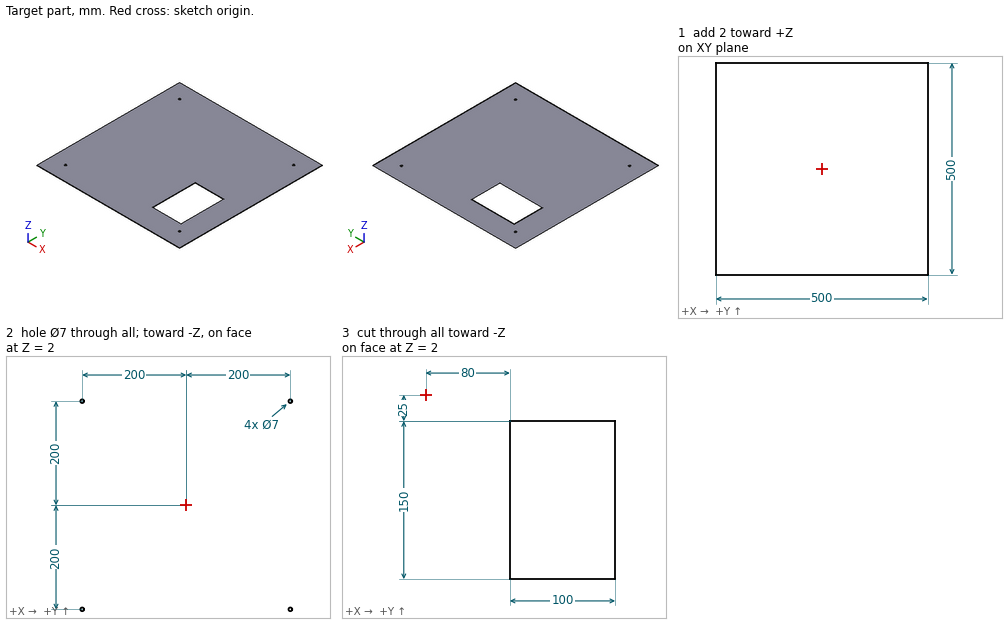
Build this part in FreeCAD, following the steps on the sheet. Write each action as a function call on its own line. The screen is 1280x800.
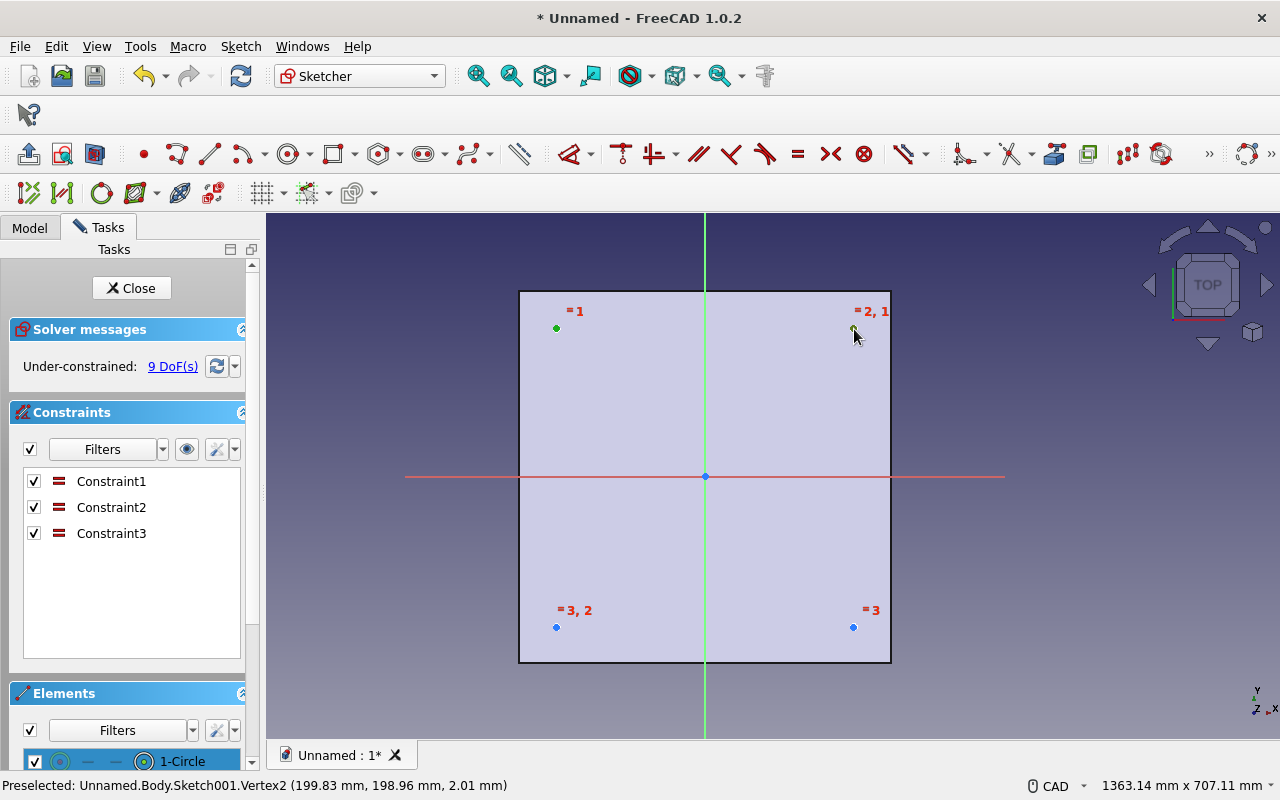
key(h)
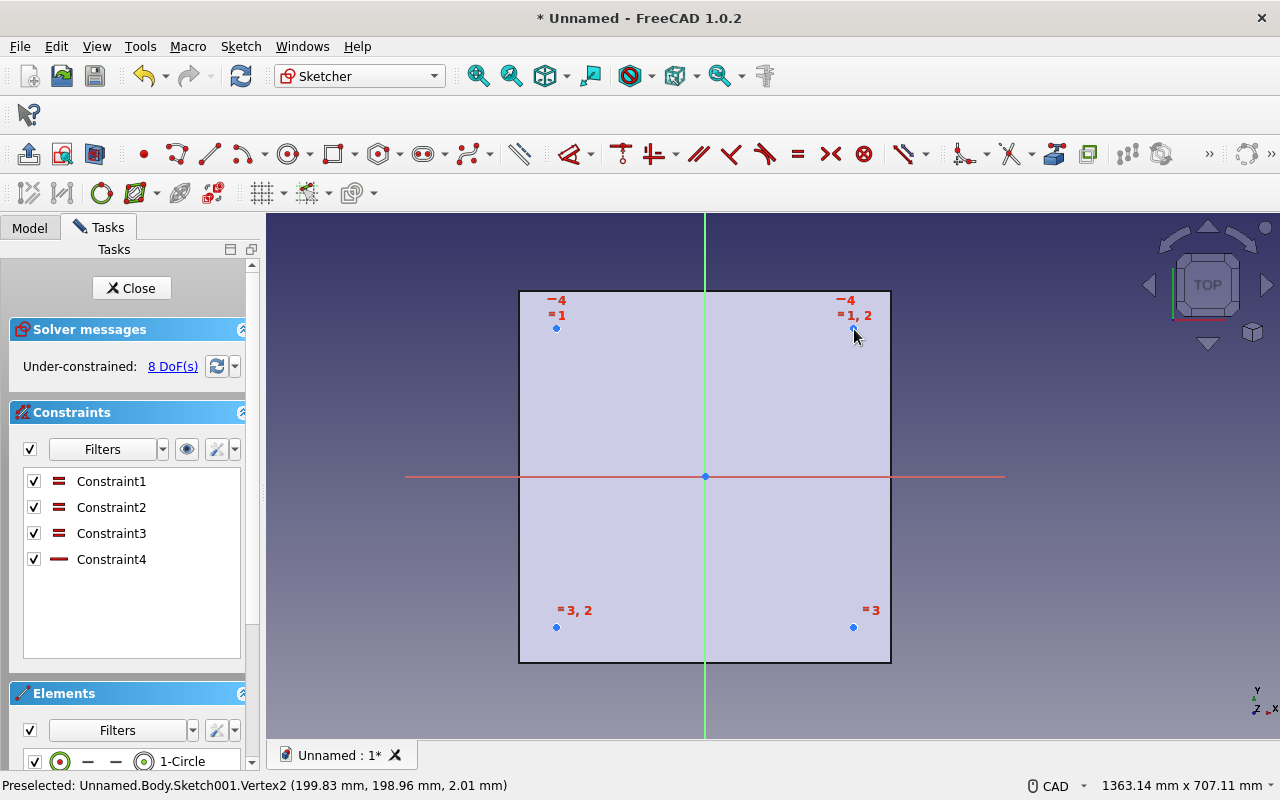
click(557, 329)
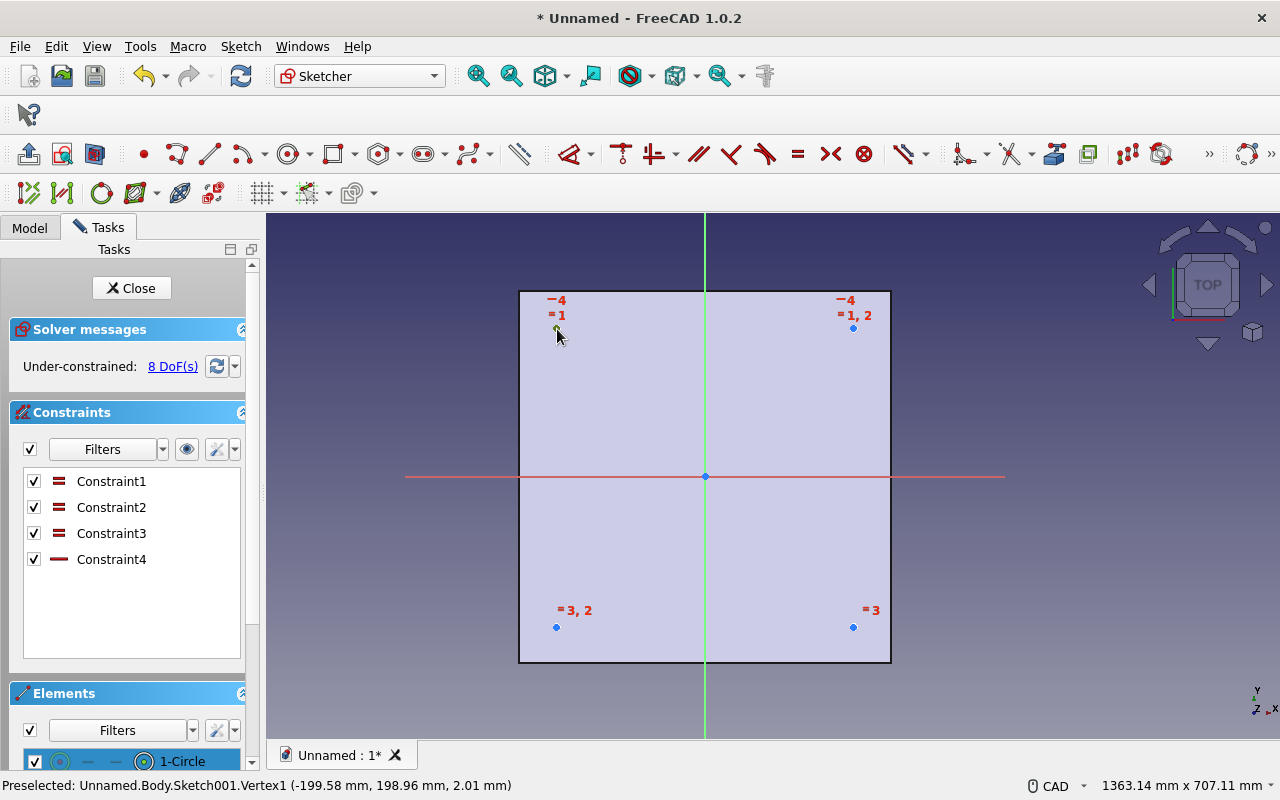
click(557, 627)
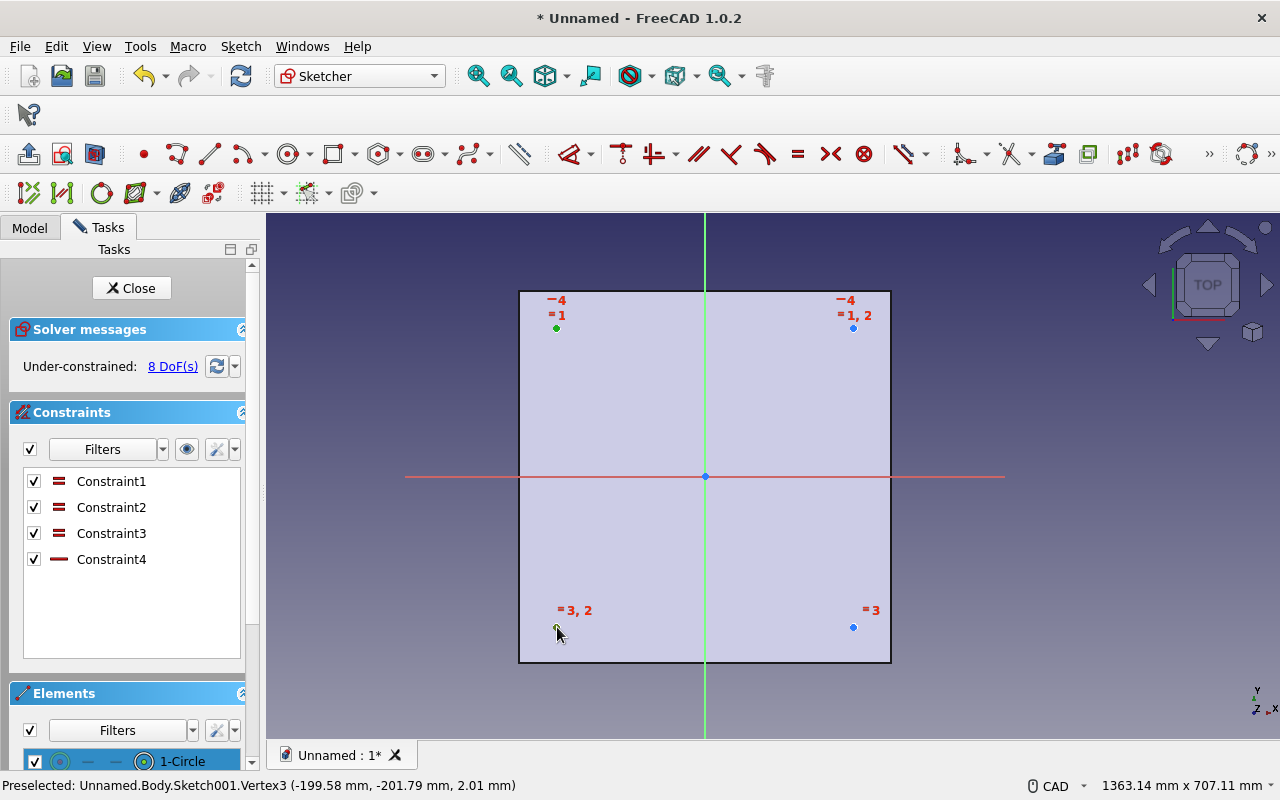
key(v)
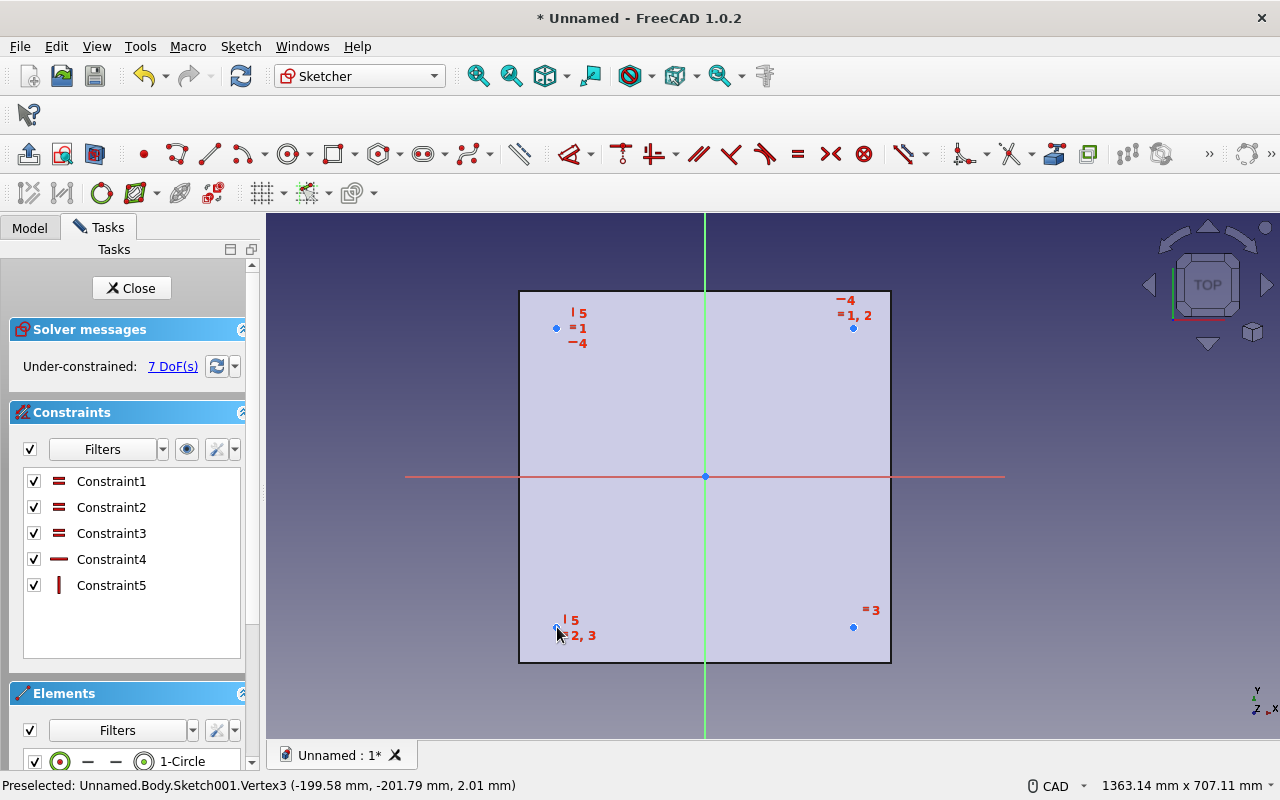
click(854, 329)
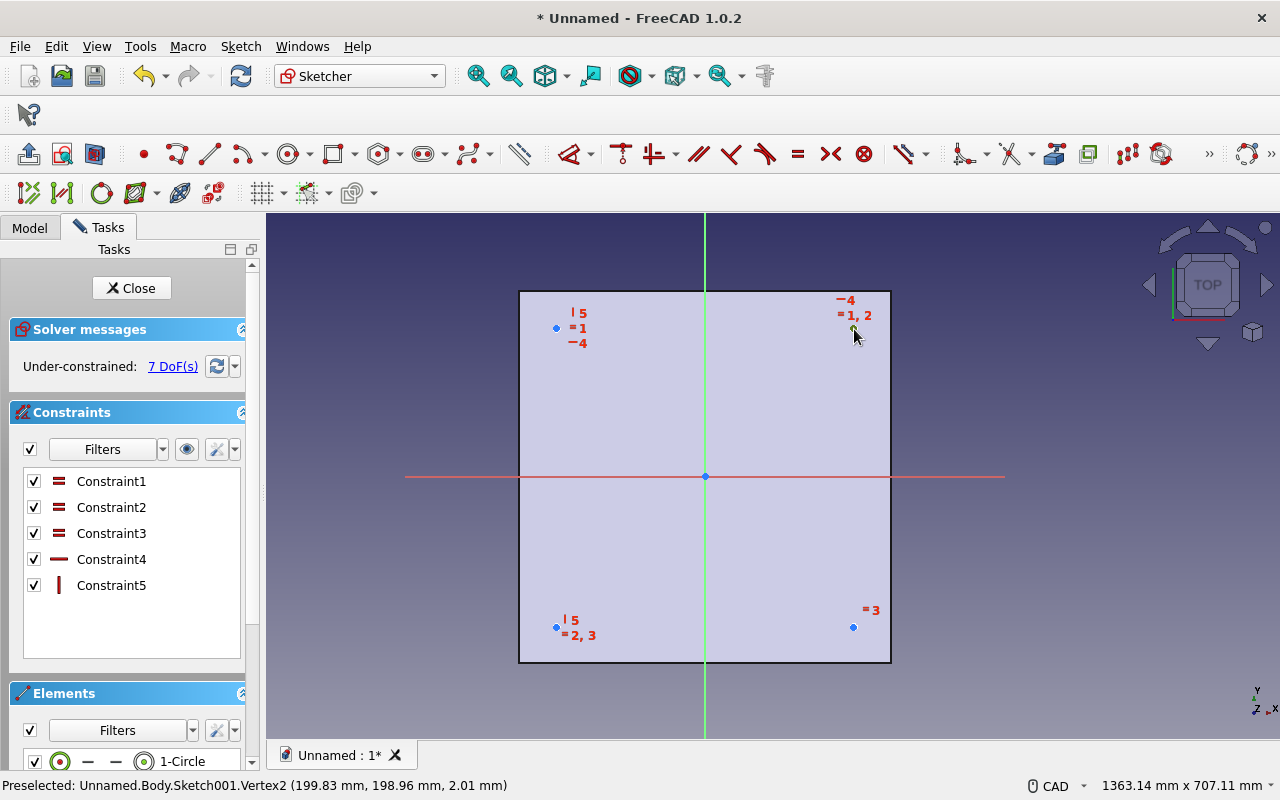
click(854, 627)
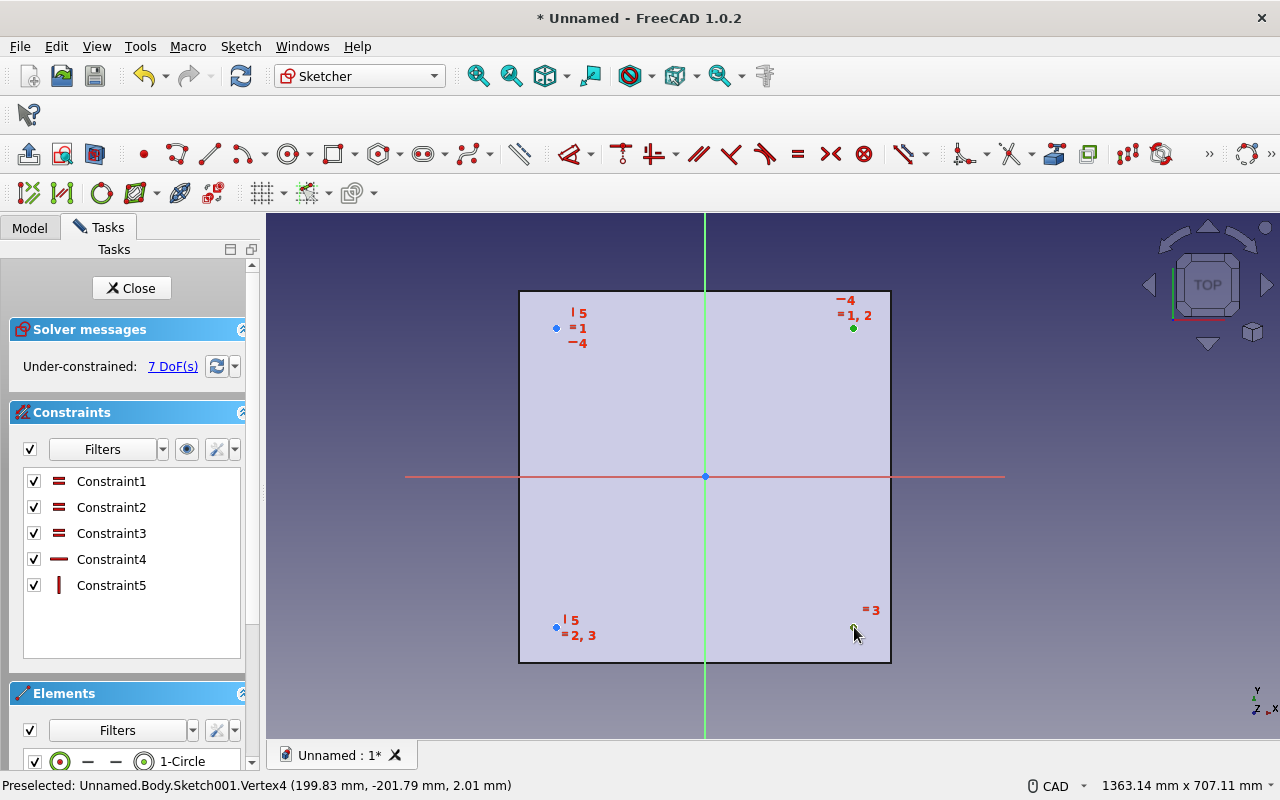
key(v)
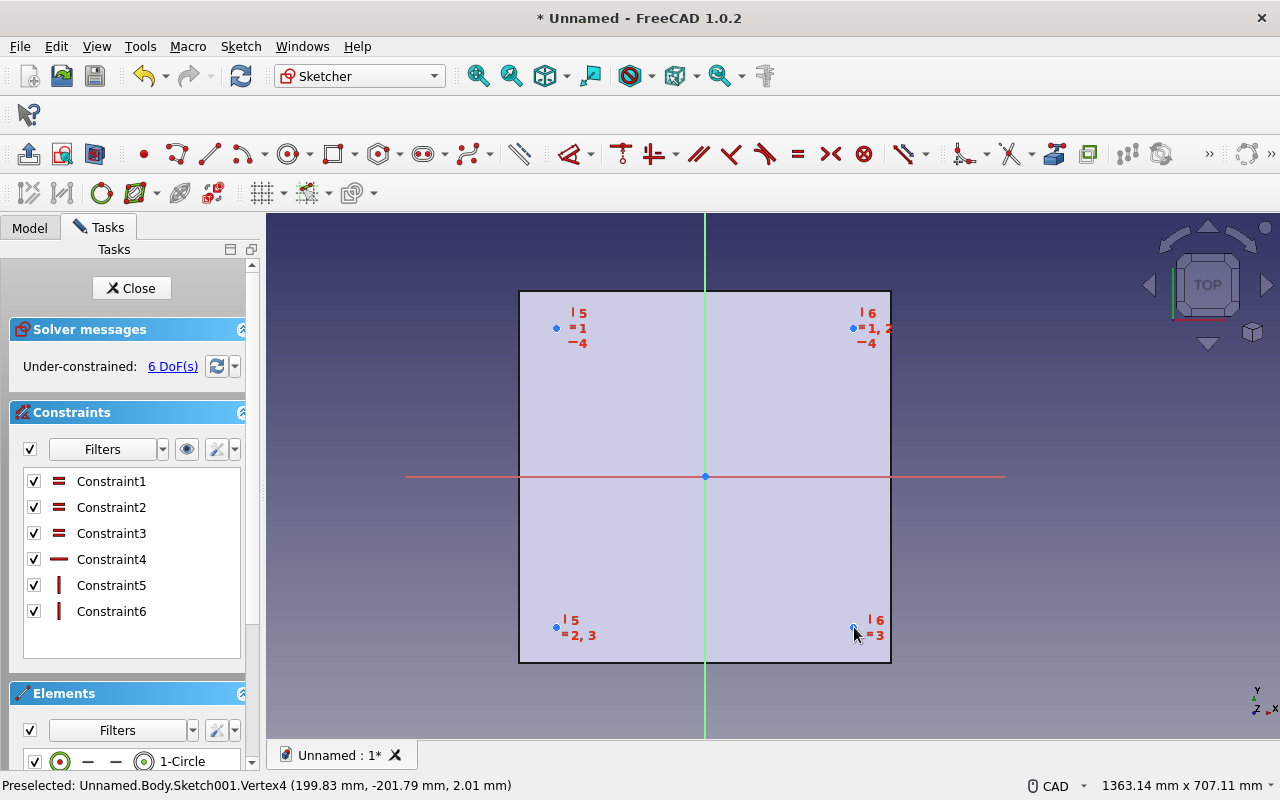
click(557, 627)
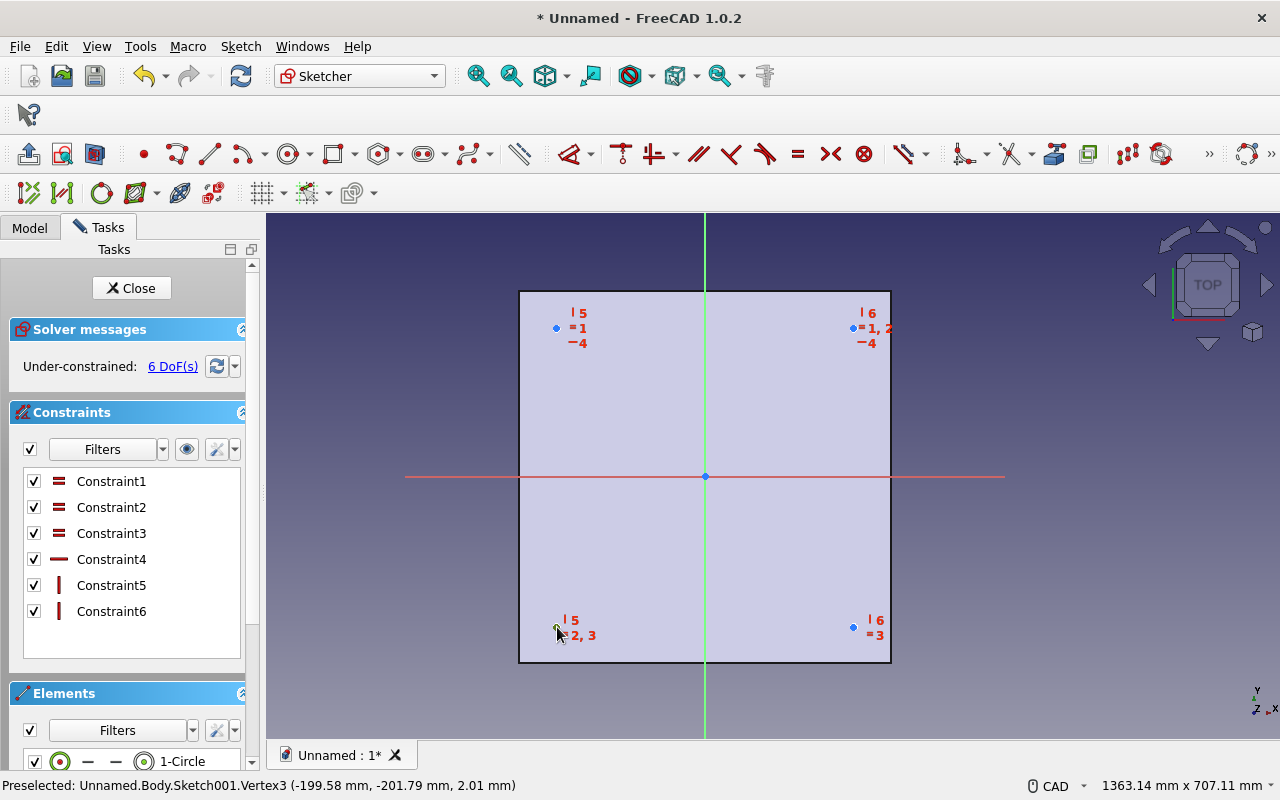
click(854, 627)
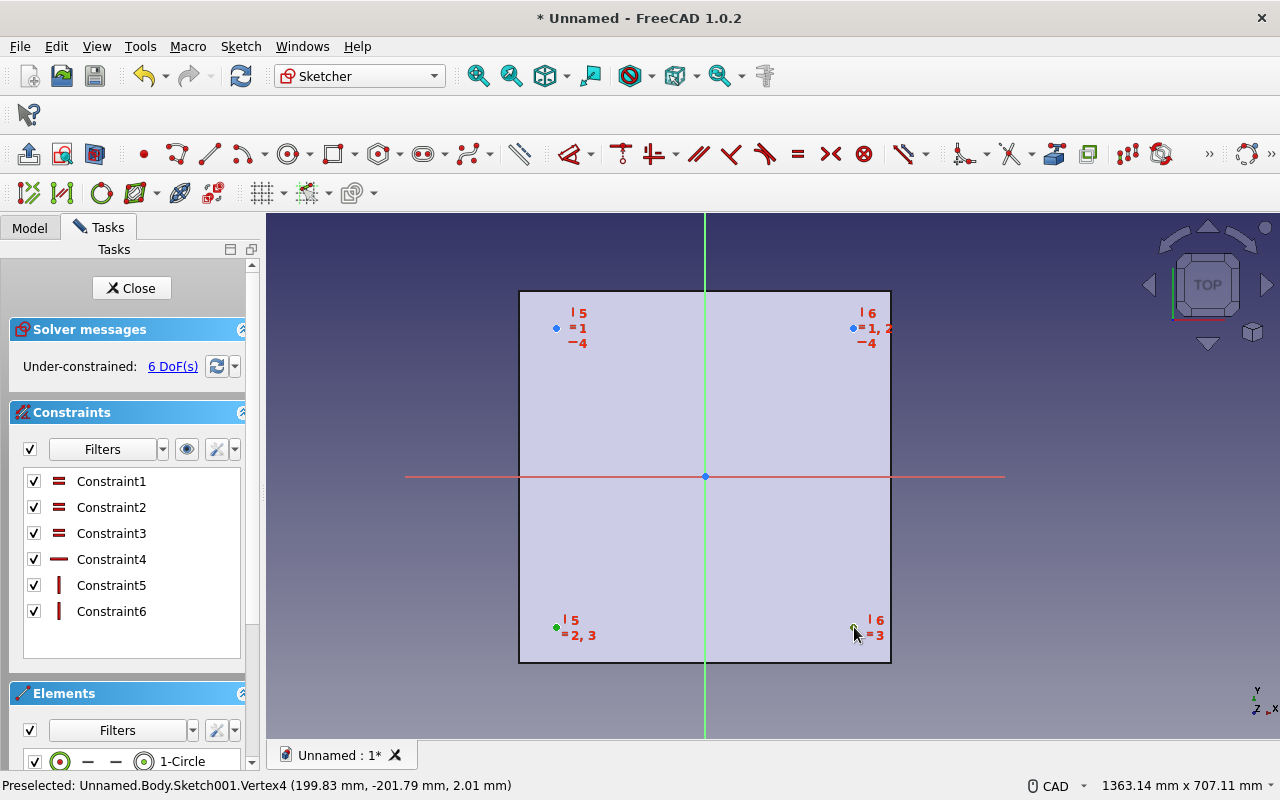
key(h)